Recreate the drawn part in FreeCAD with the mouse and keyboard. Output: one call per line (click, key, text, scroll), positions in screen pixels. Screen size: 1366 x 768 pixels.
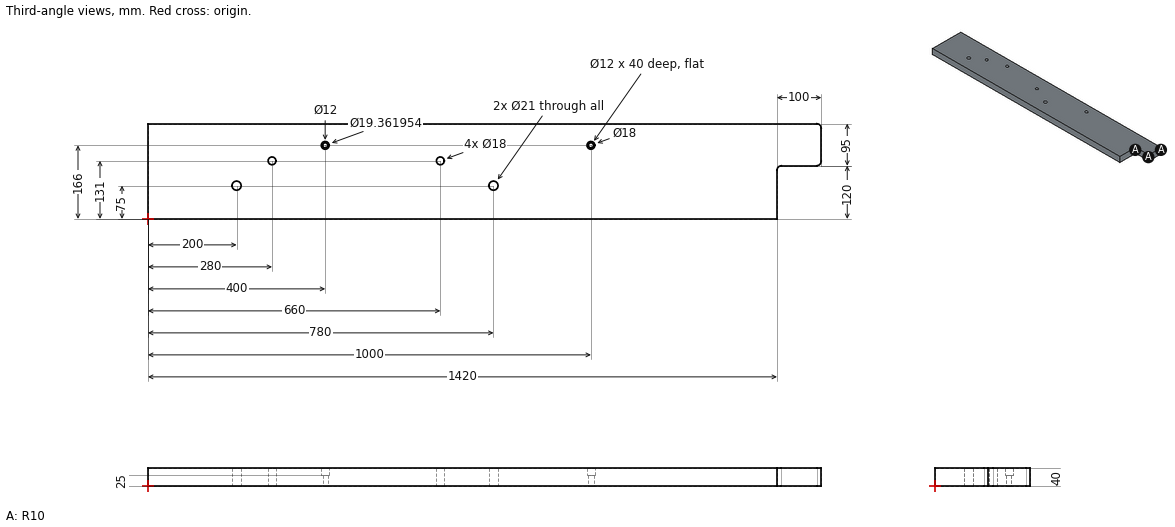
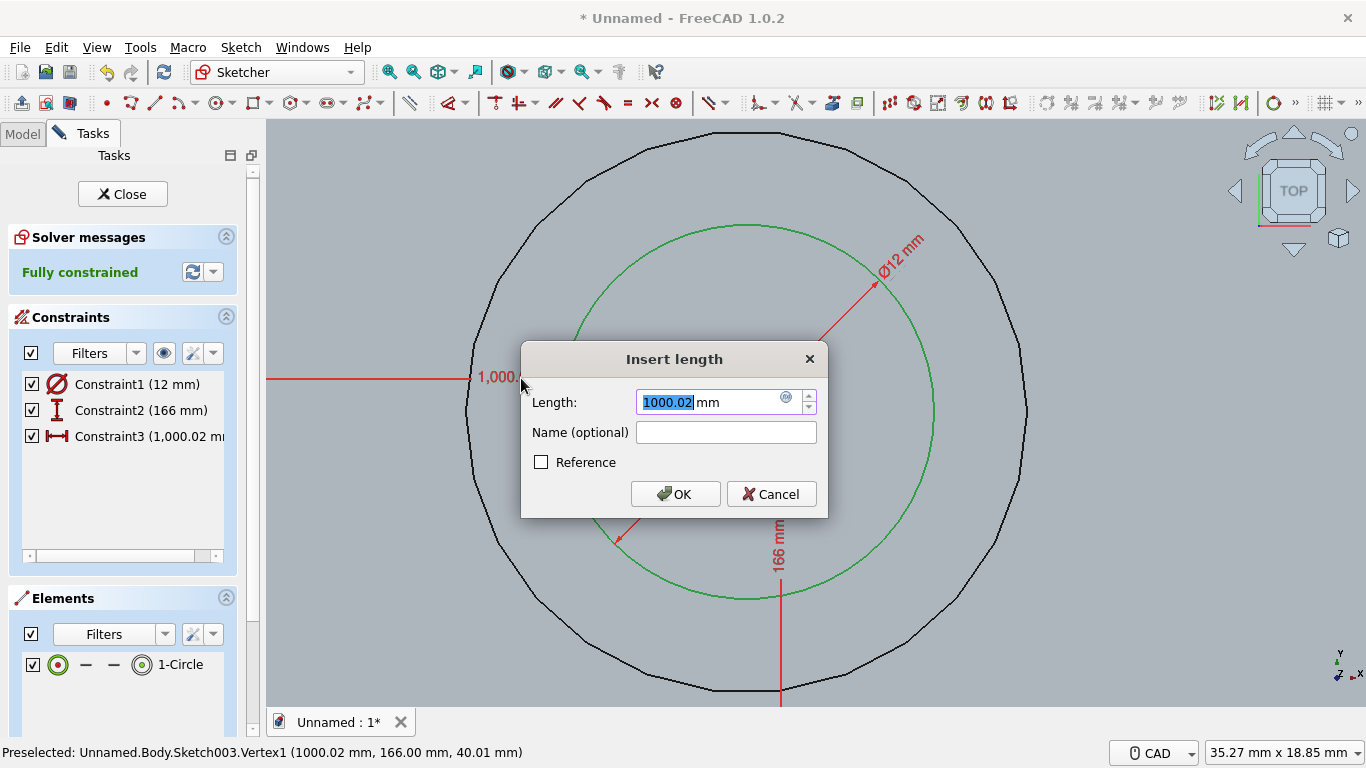
text(1000)
key(Return)
key(Escape)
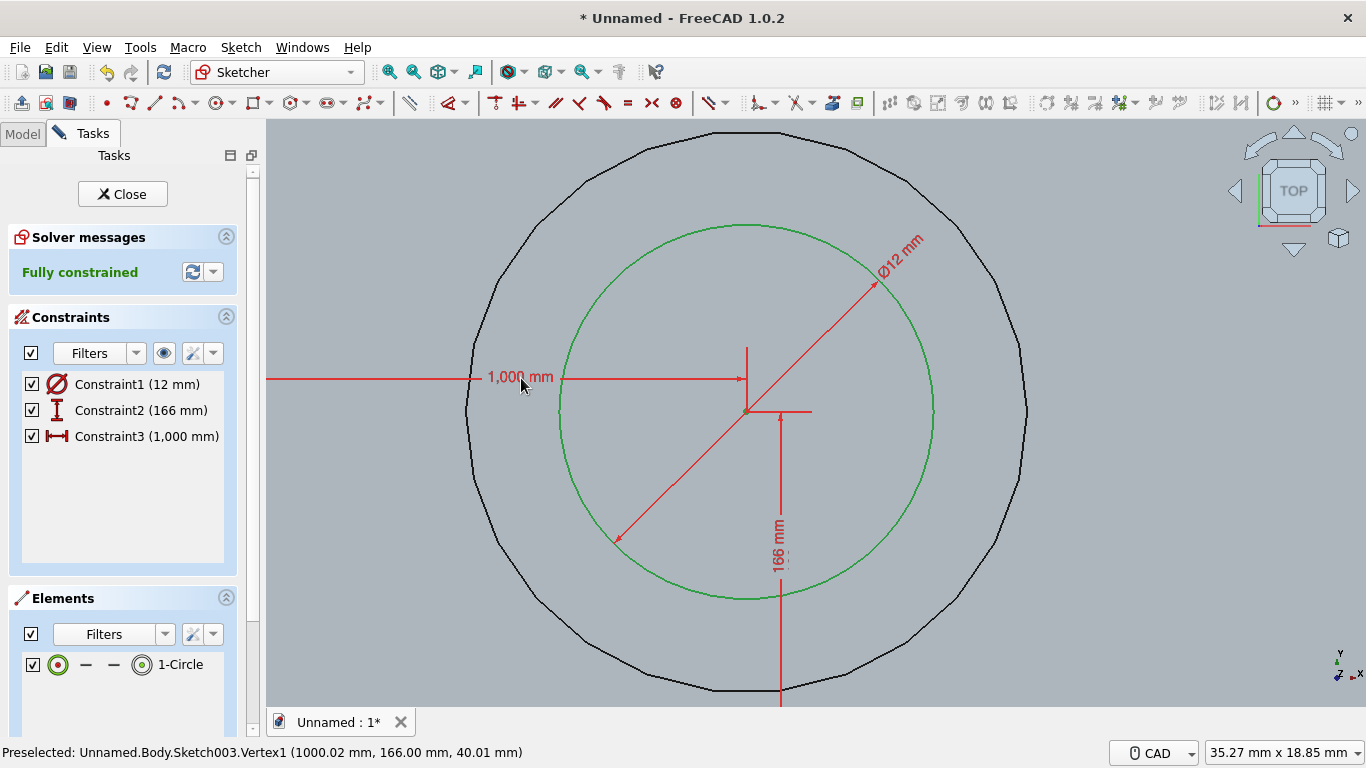
click(123, 194)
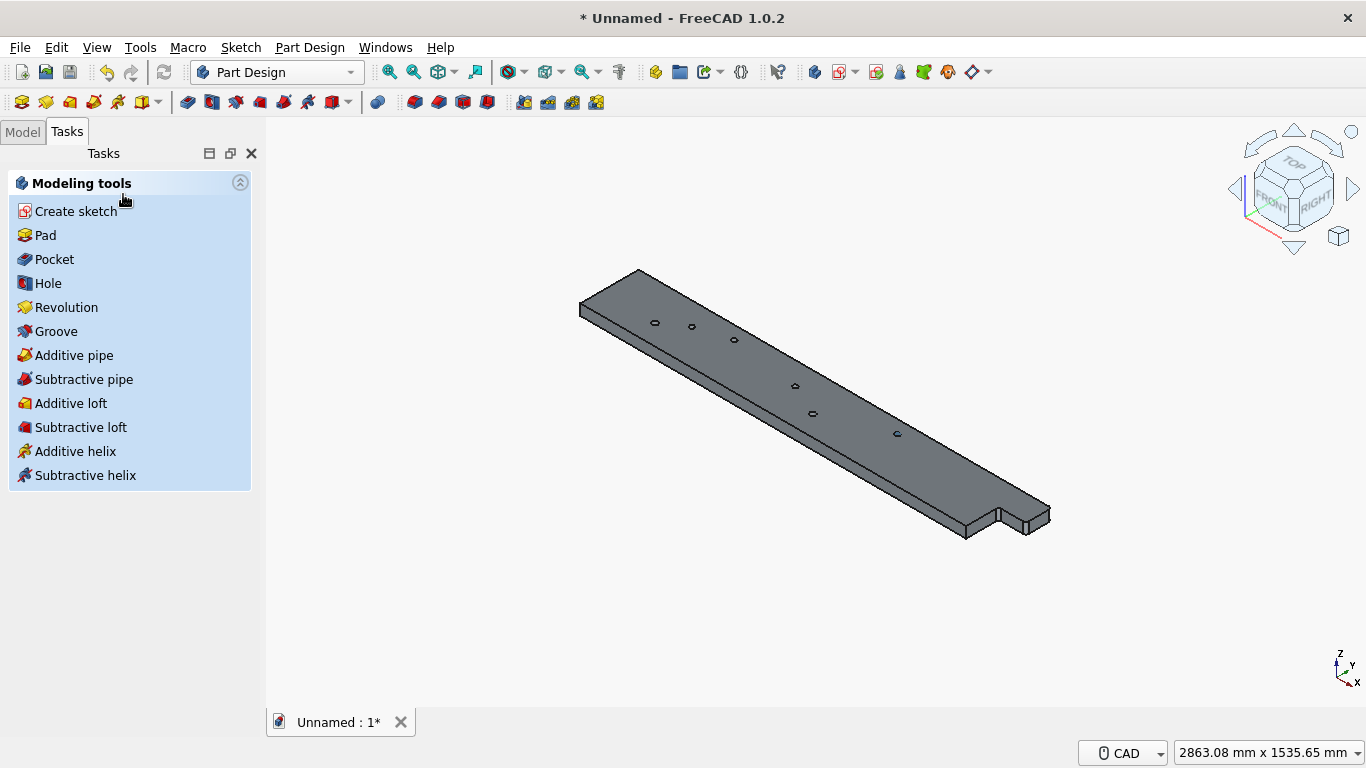
click(212, 102)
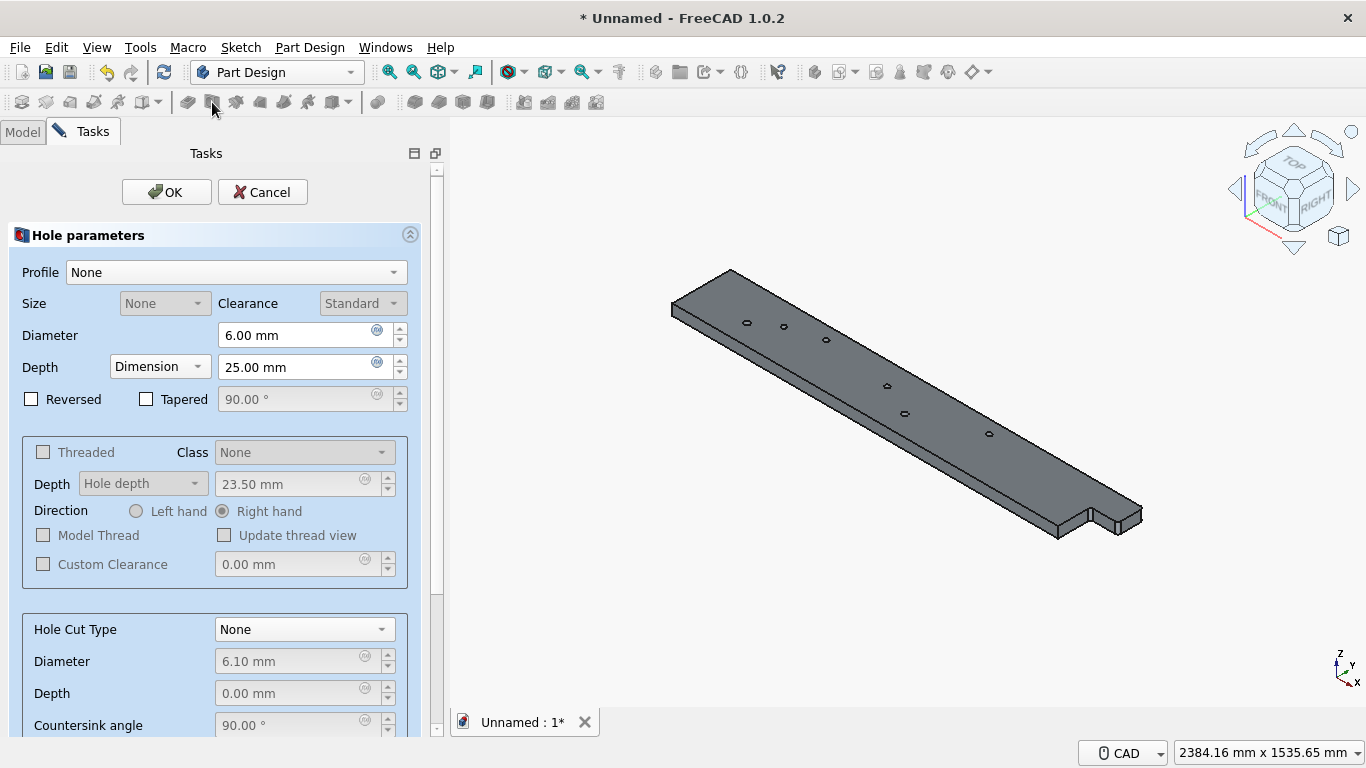
triple_click(305, 335)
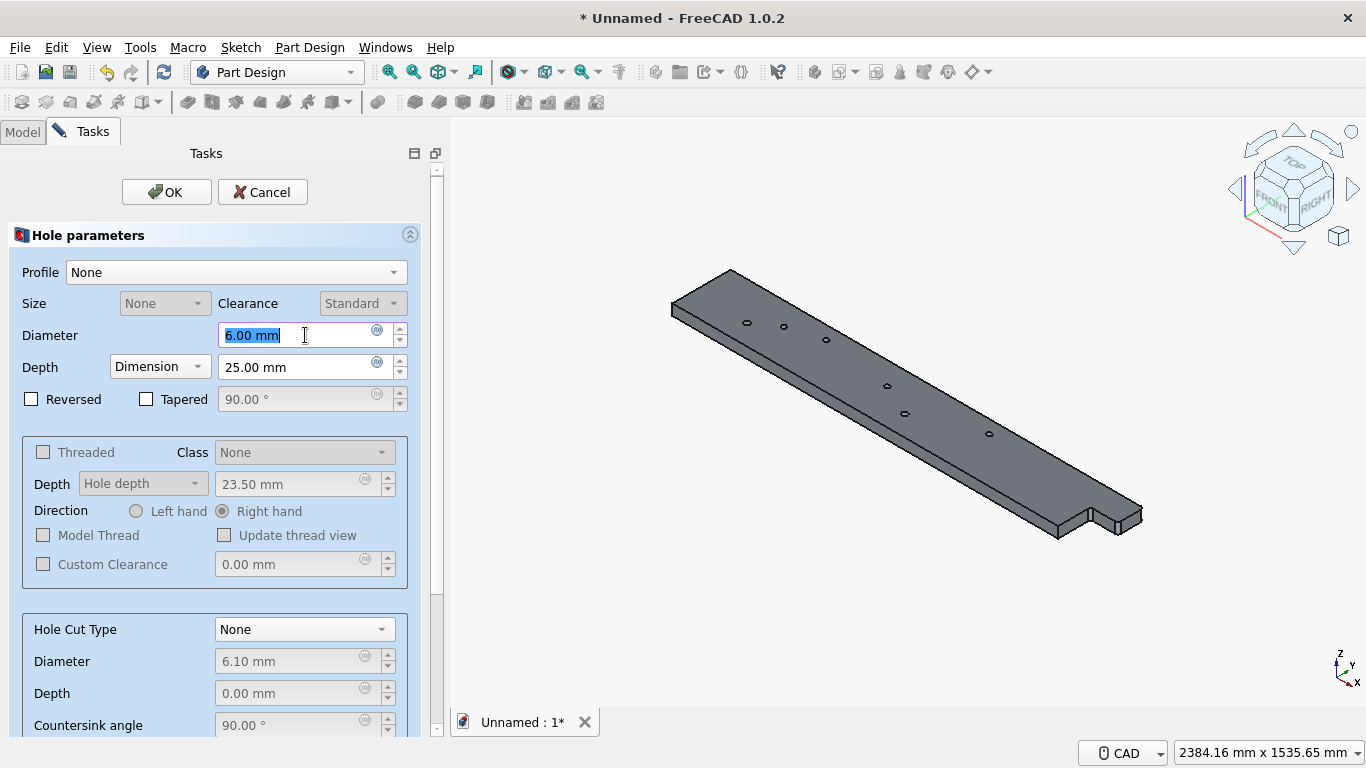
text(12)
key(Tab)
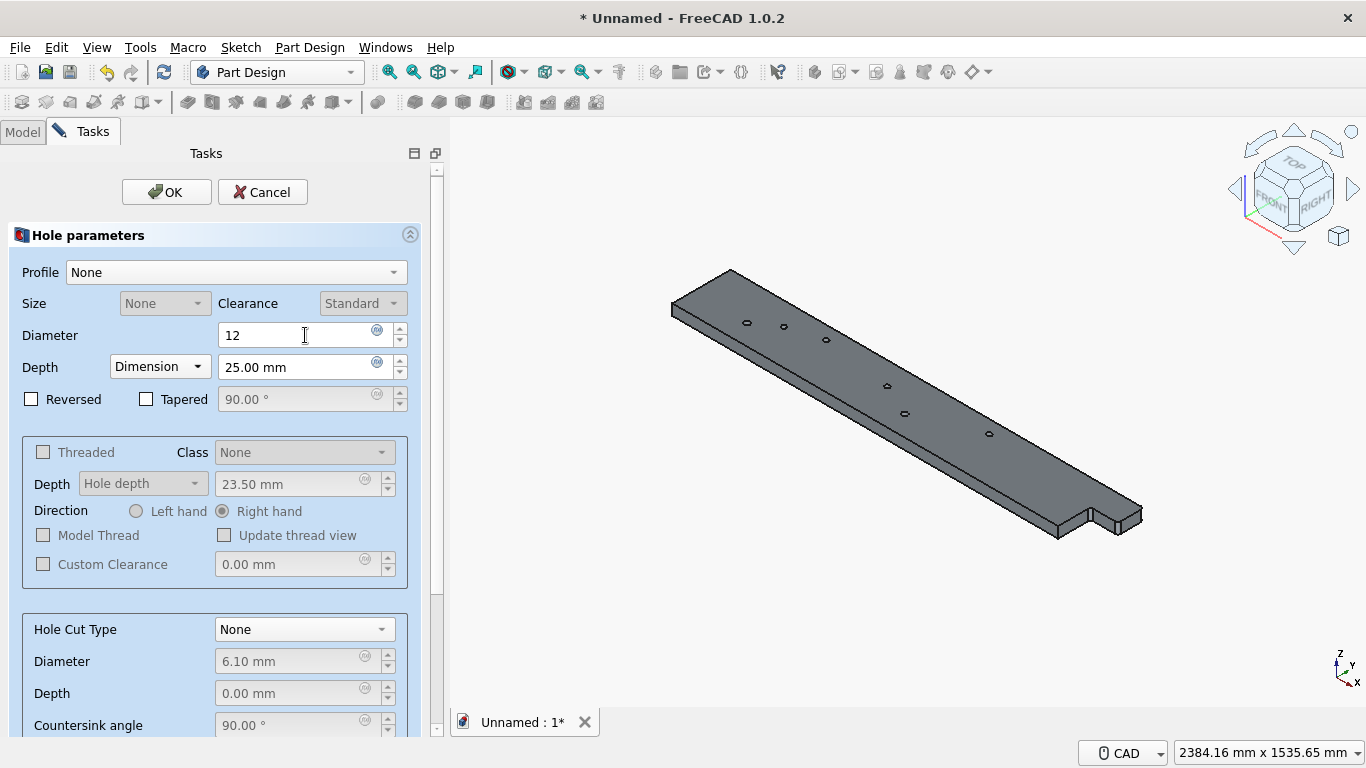
triple_click(305, 367)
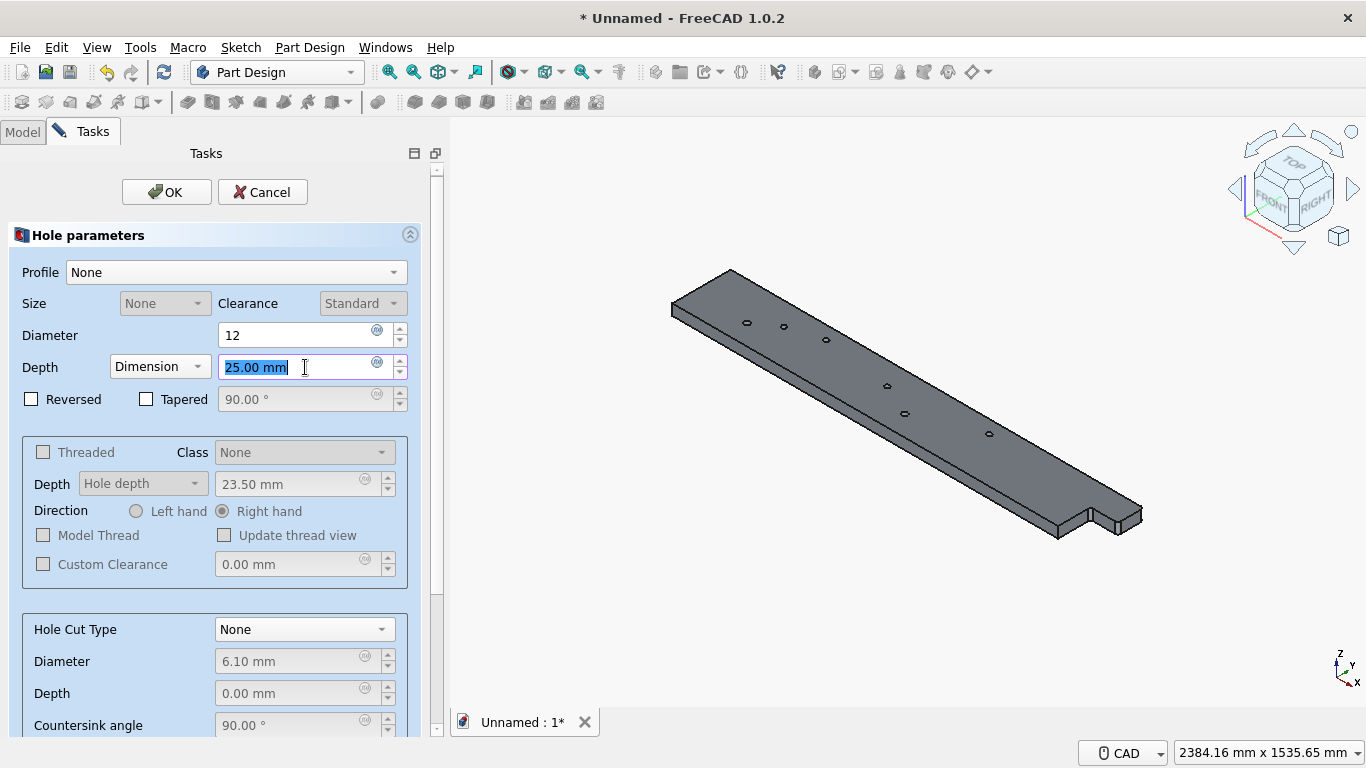
text(40)
key(Tab)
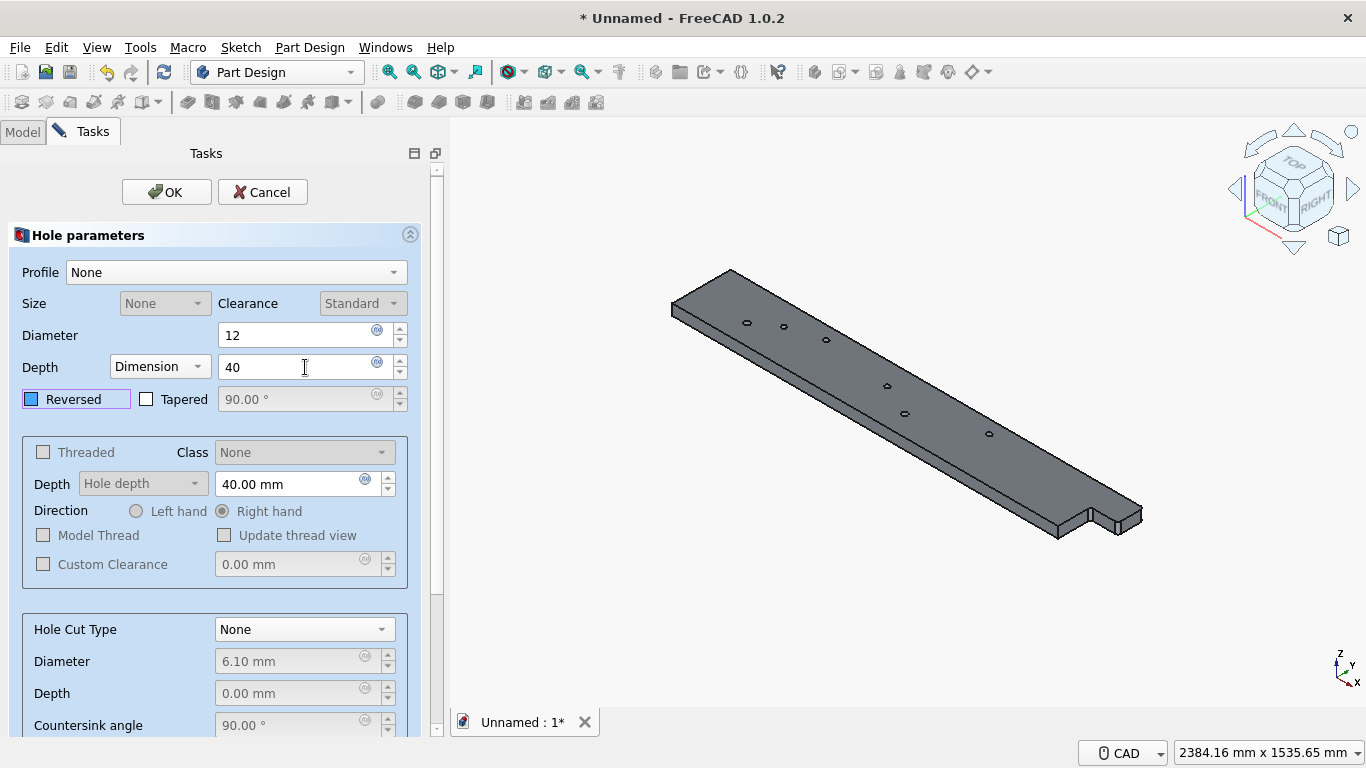
scroll(437, 450, down, 3)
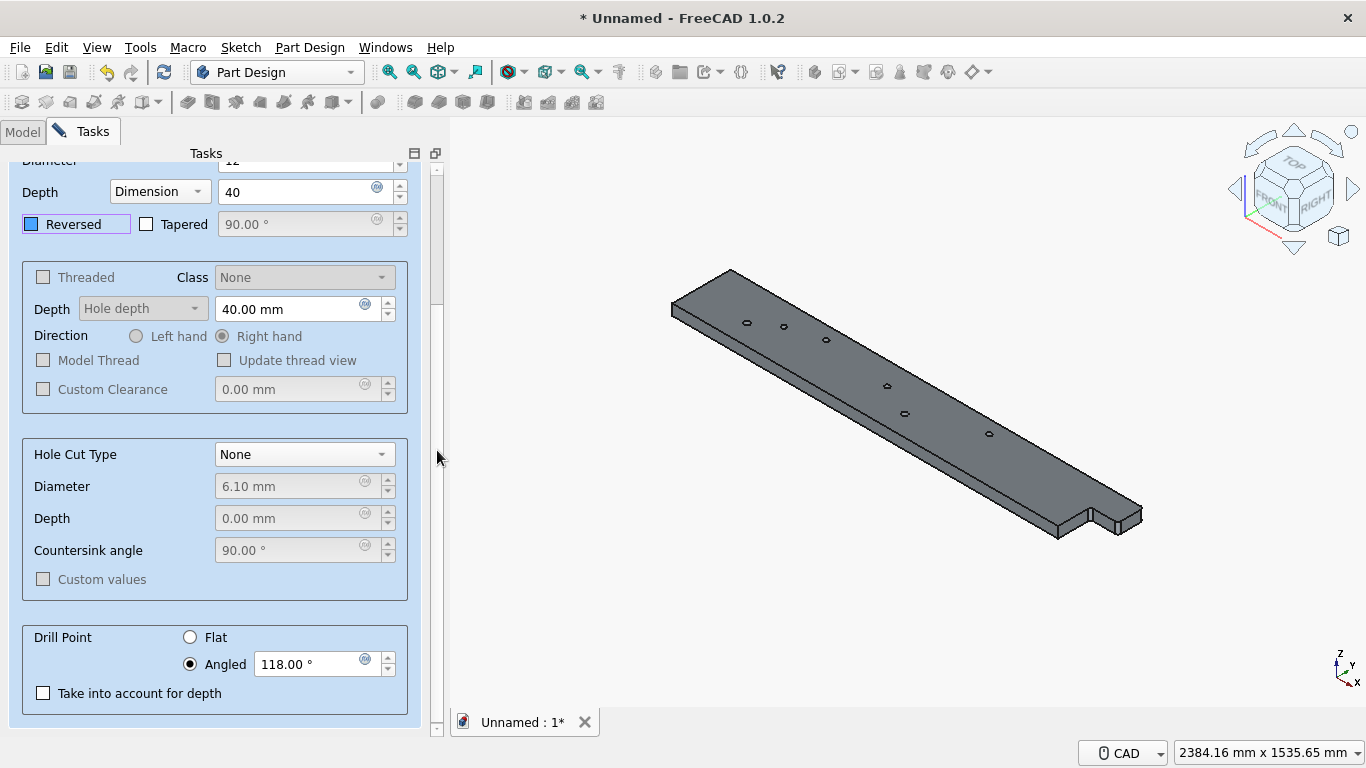
click(191, 637)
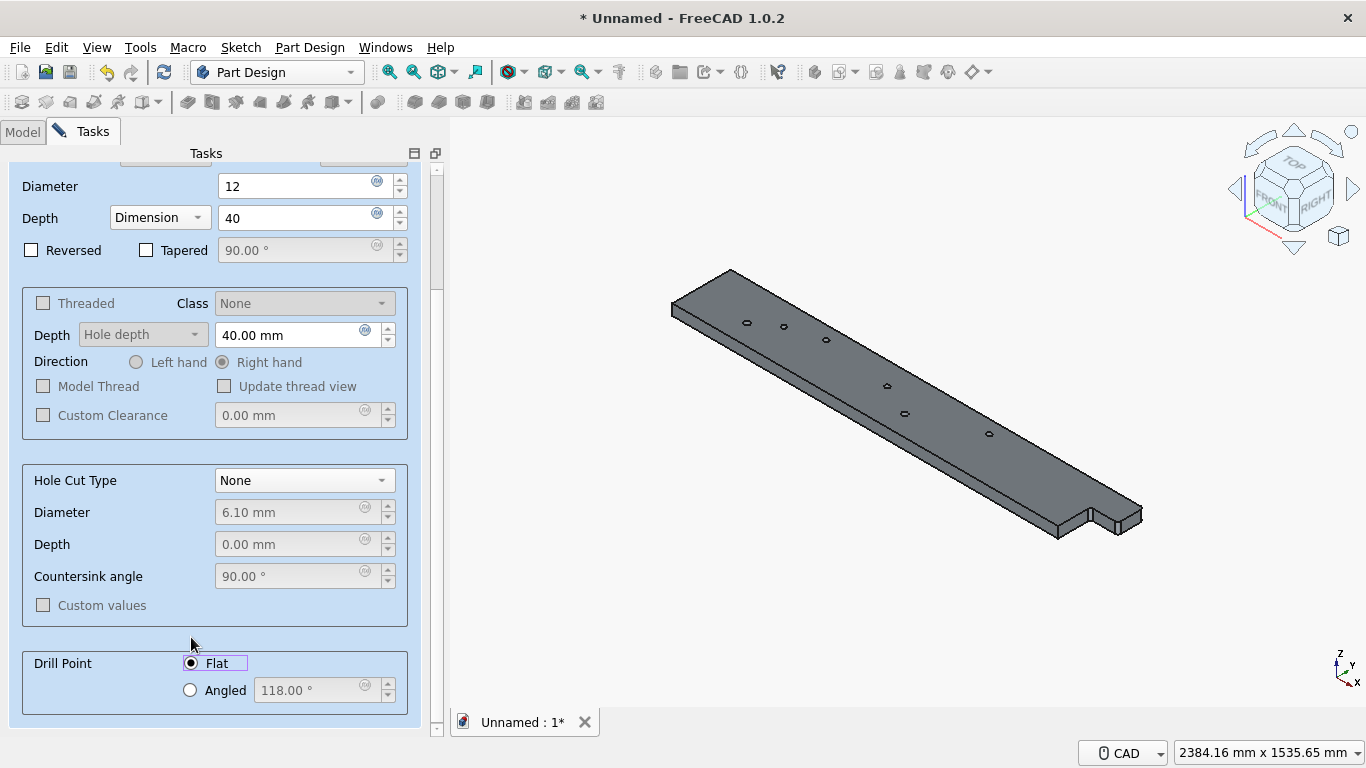
scroll(437, 450, up, 4)